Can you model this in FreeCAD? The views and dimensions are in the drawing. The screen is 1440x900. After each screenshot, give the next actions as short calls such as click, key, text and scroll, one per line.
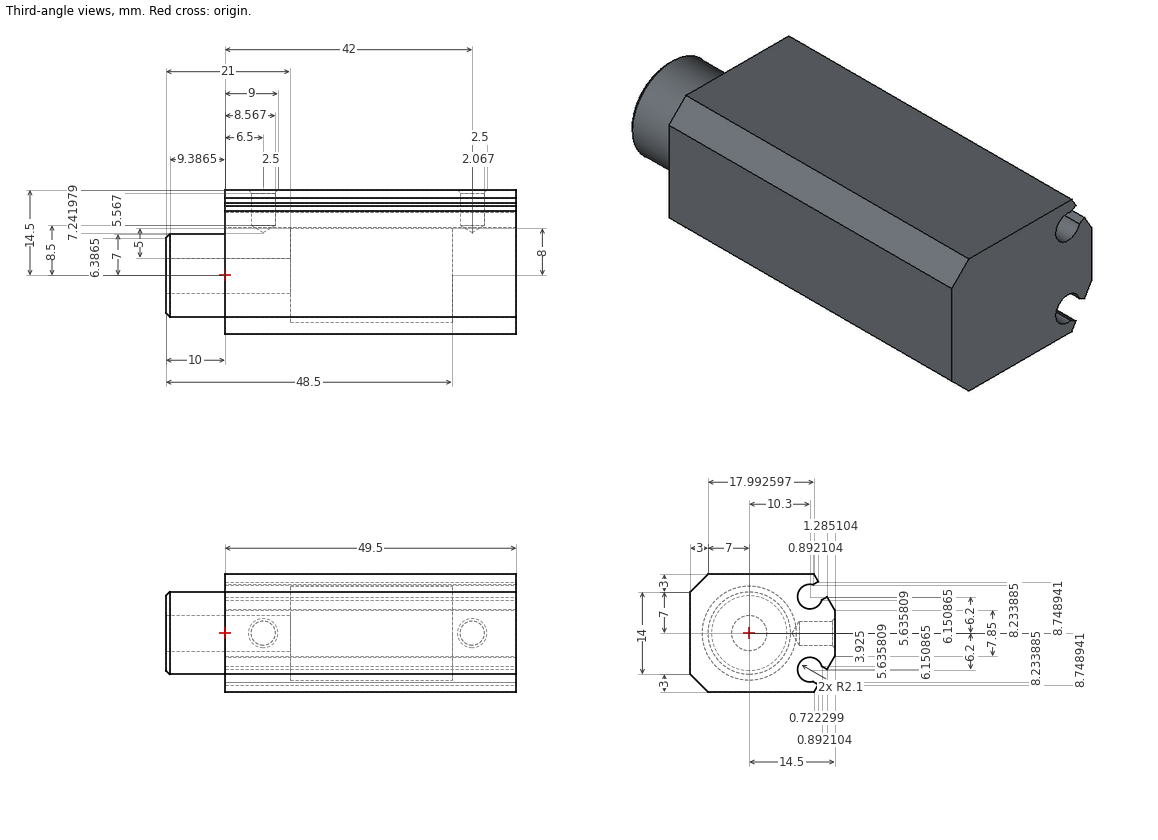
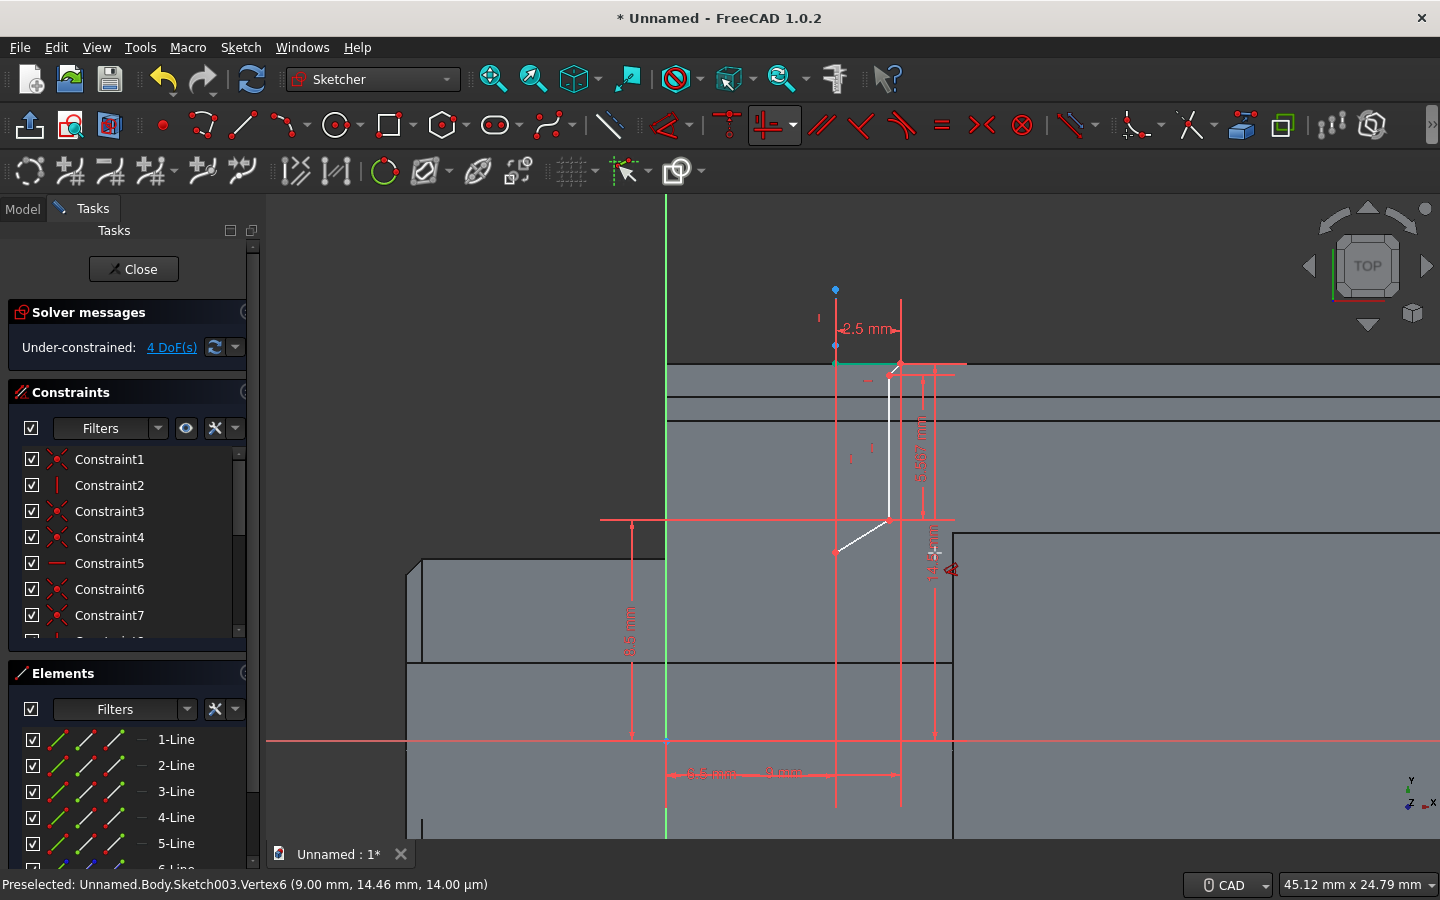
click(889, 520)
click(856, 775)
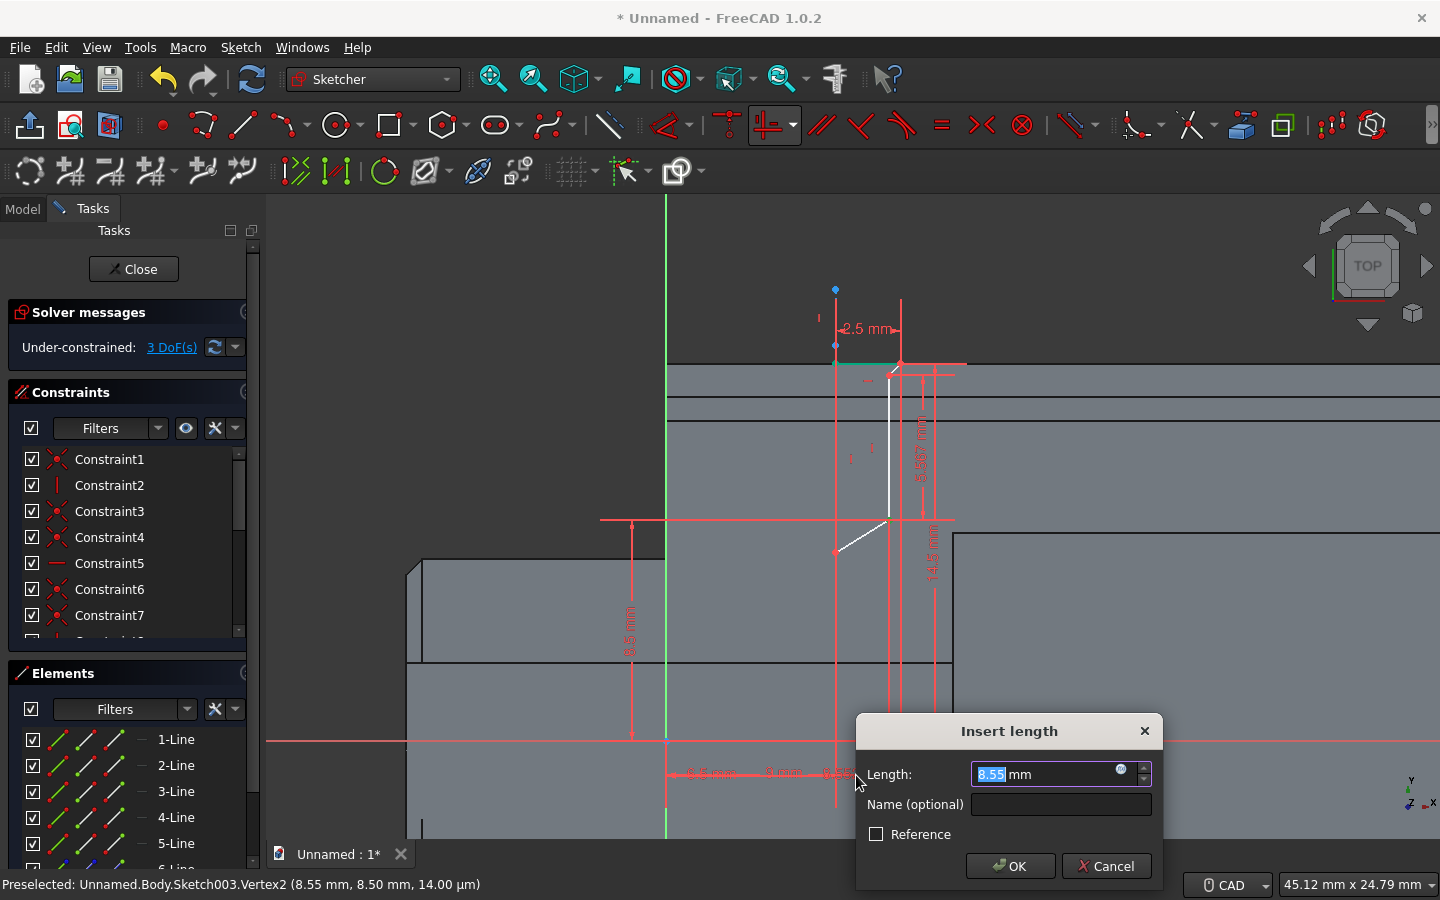
text(8.567)
key(Return)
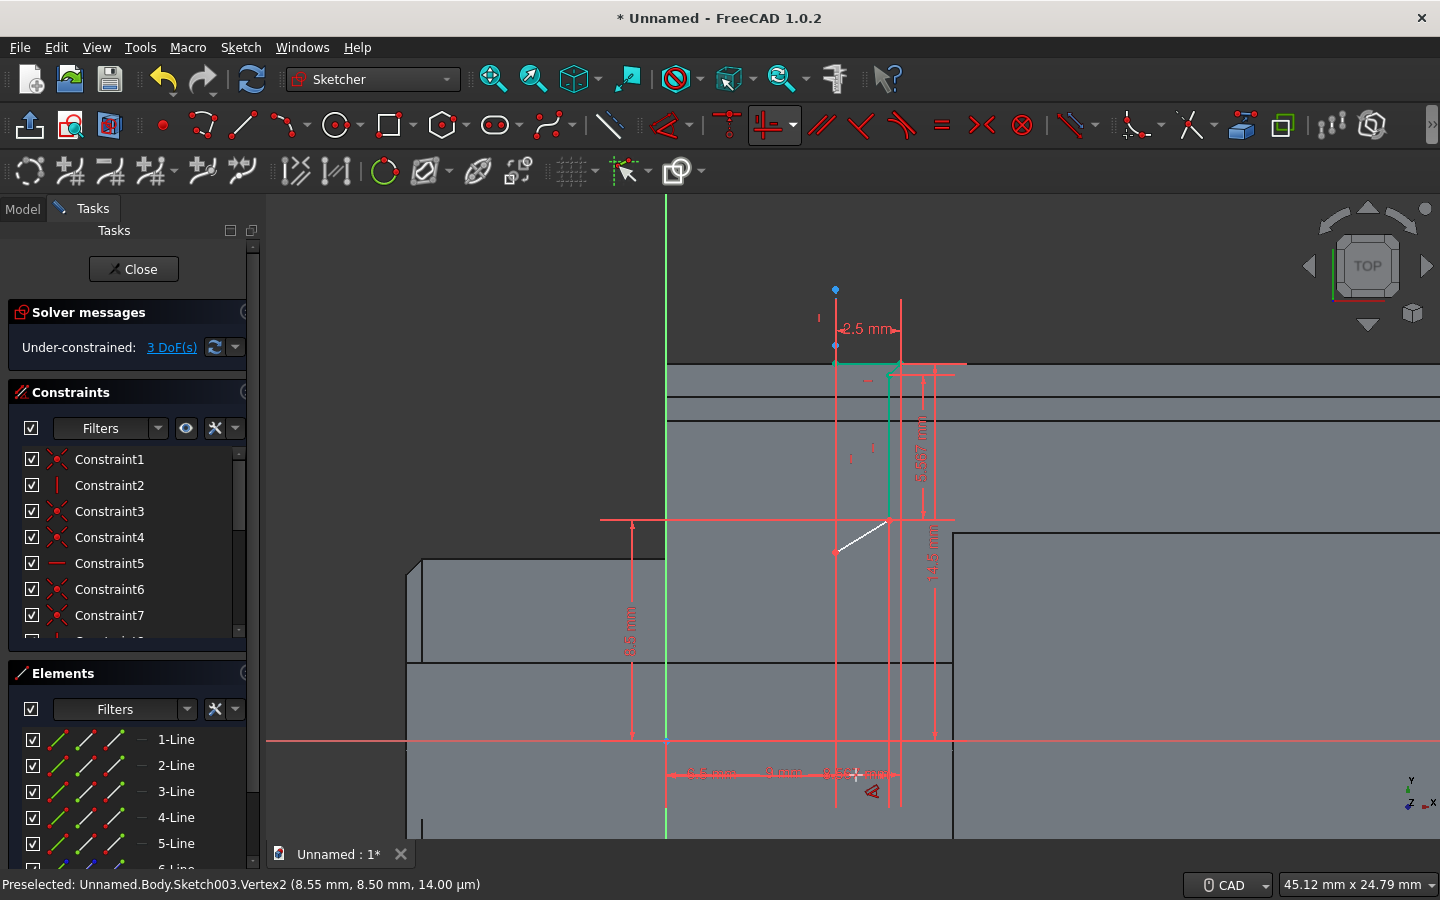
click(836, 421)
click(870, 415)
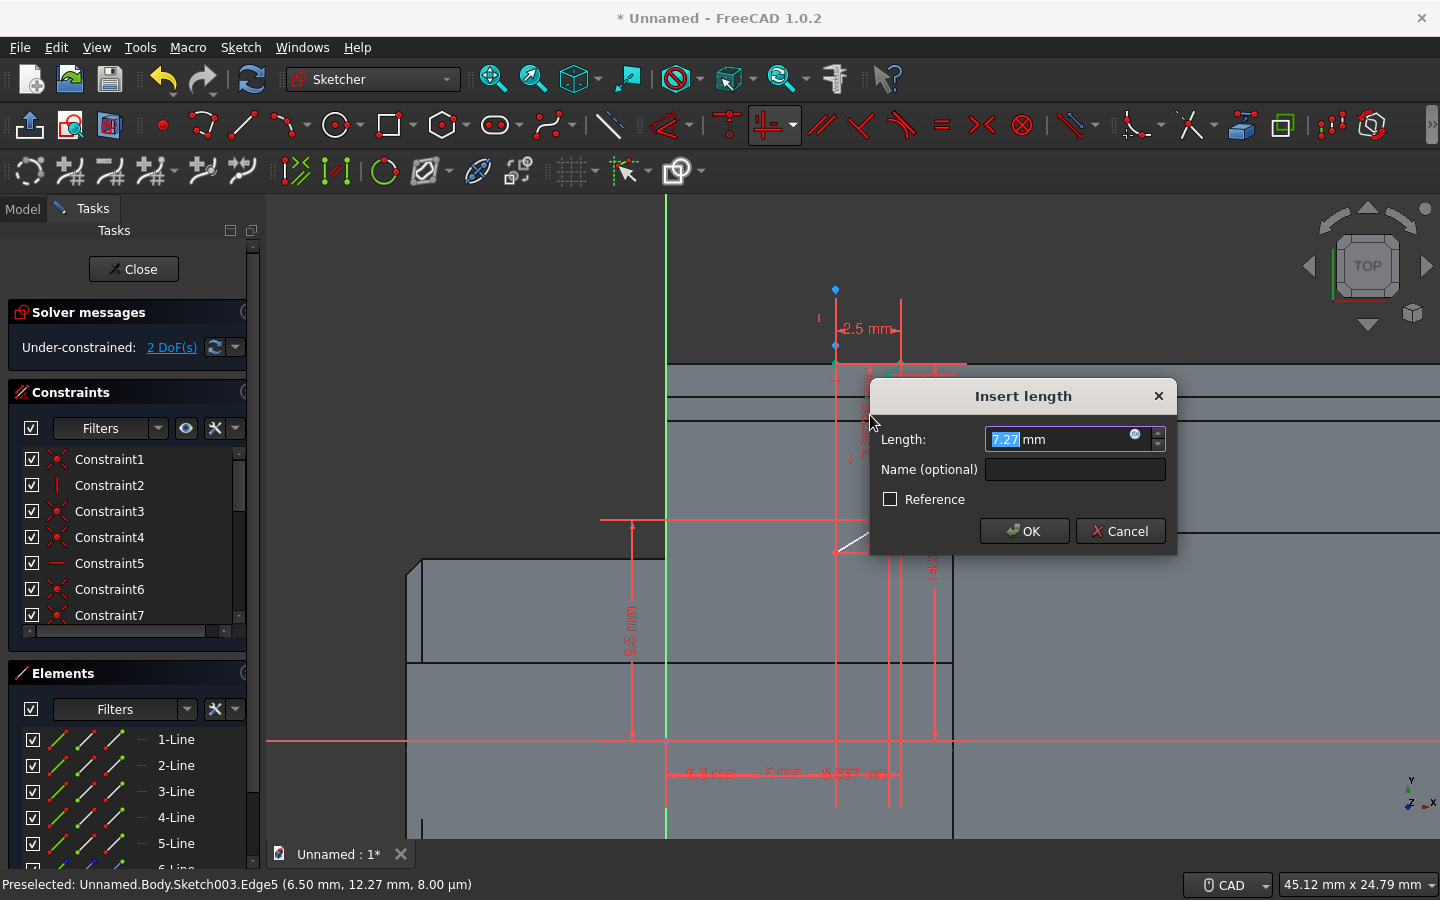
text(7.241979)
key(Return)
key(Escape)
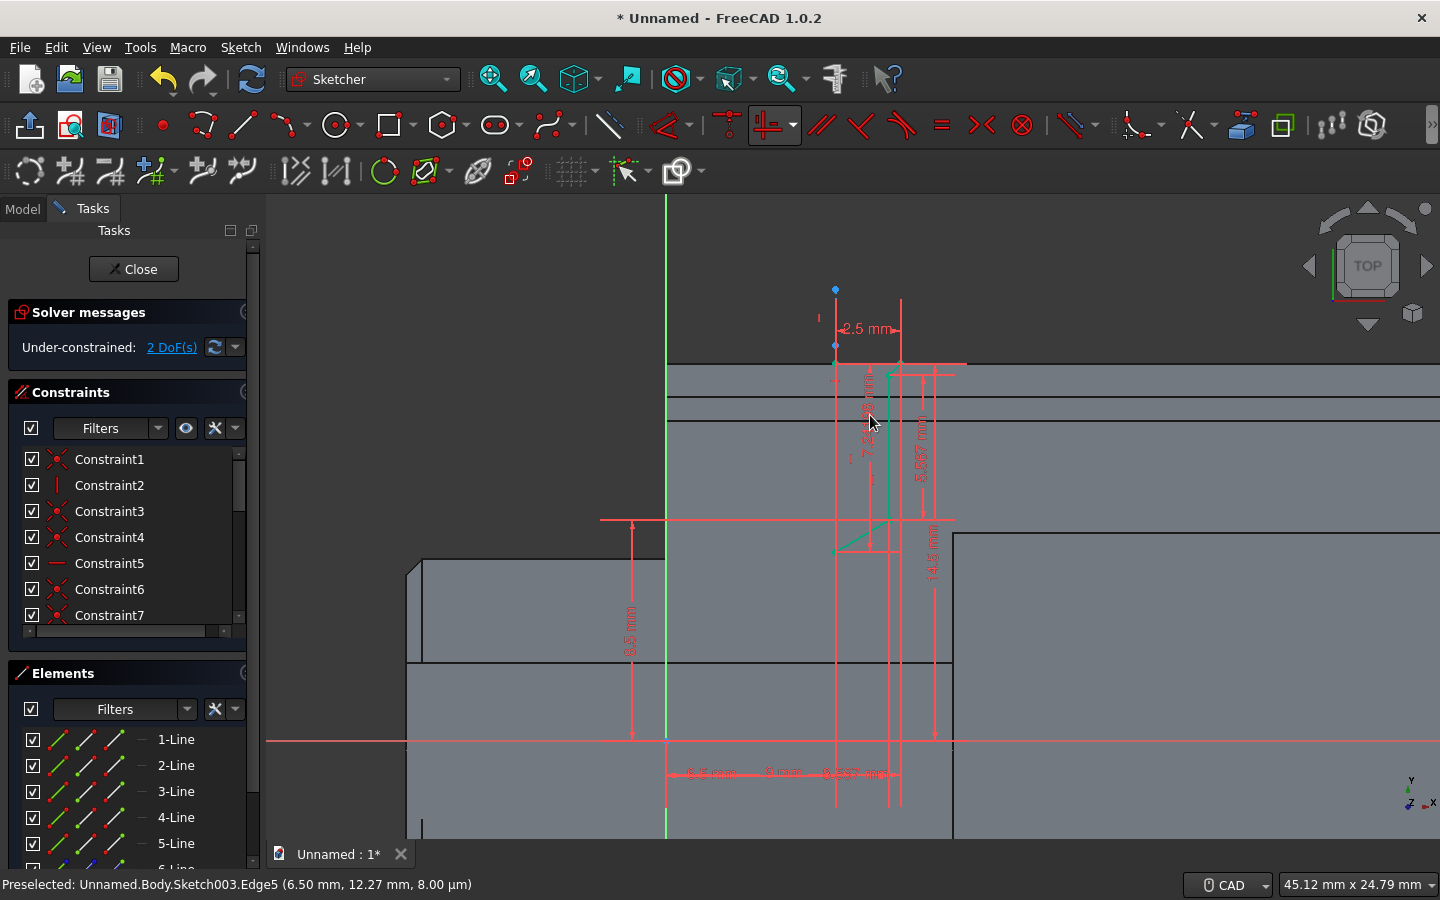
click(134, 269)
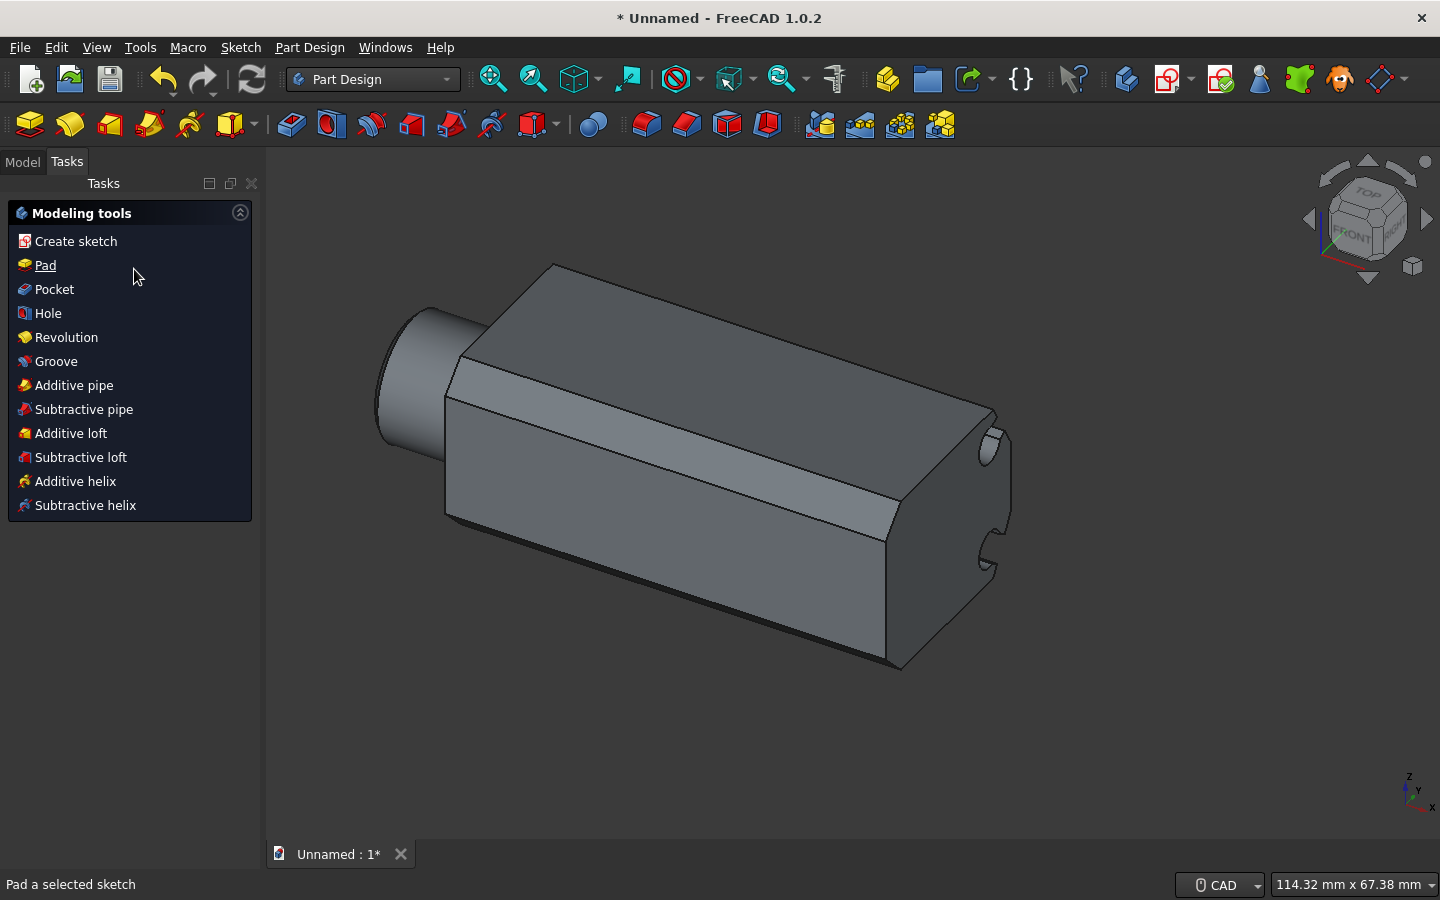
click(372, 124)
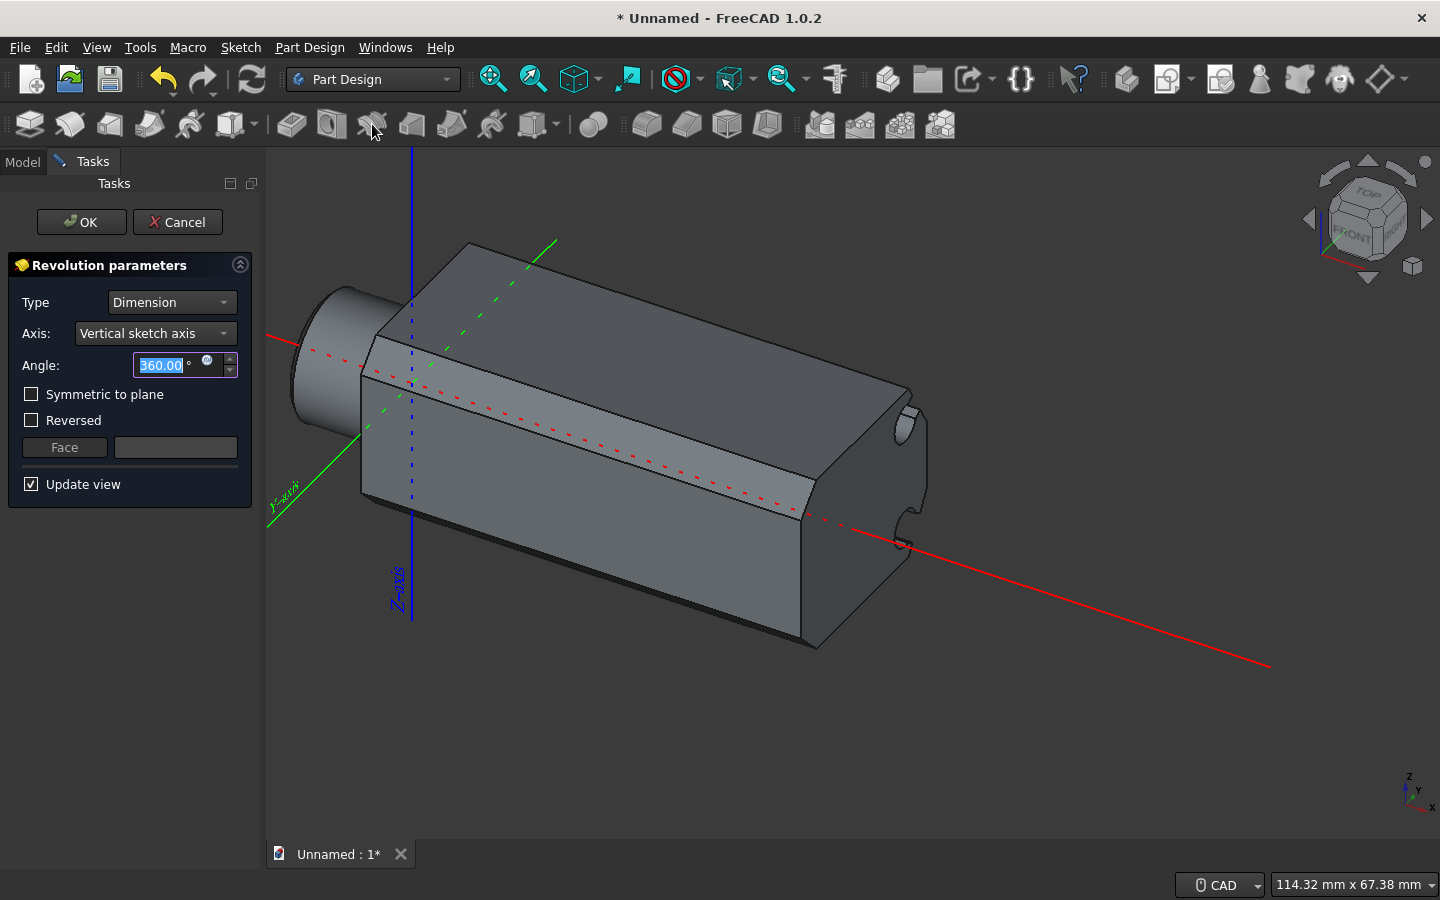
click(156, 334)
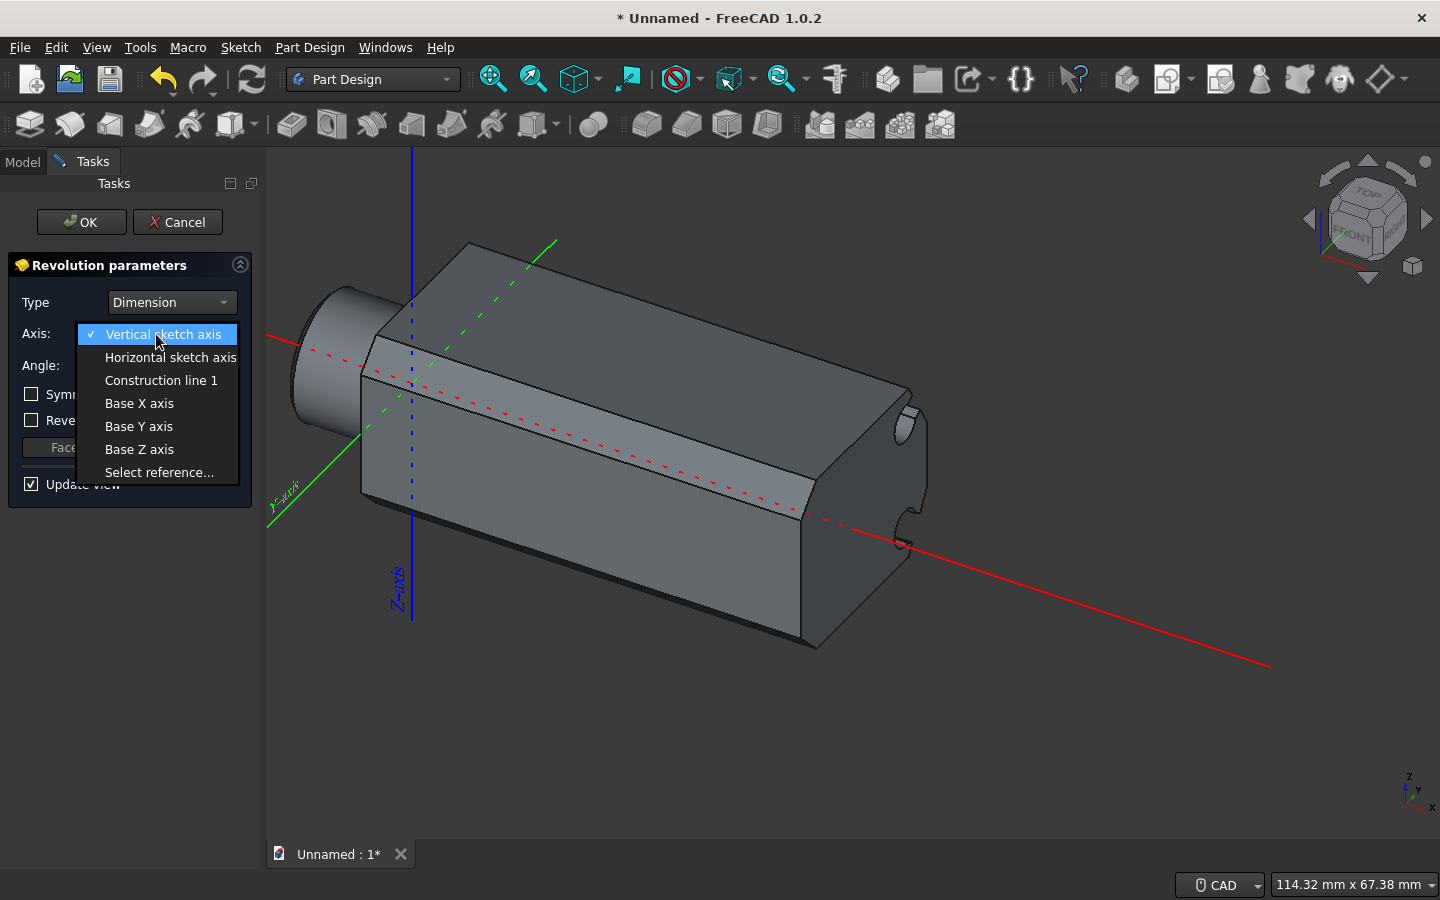
click(156, 380)